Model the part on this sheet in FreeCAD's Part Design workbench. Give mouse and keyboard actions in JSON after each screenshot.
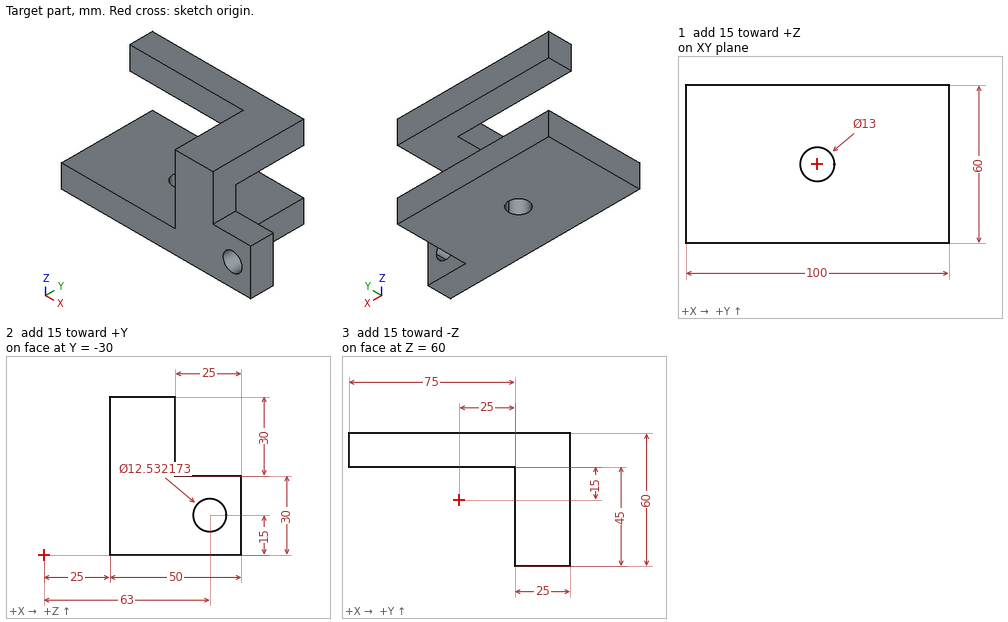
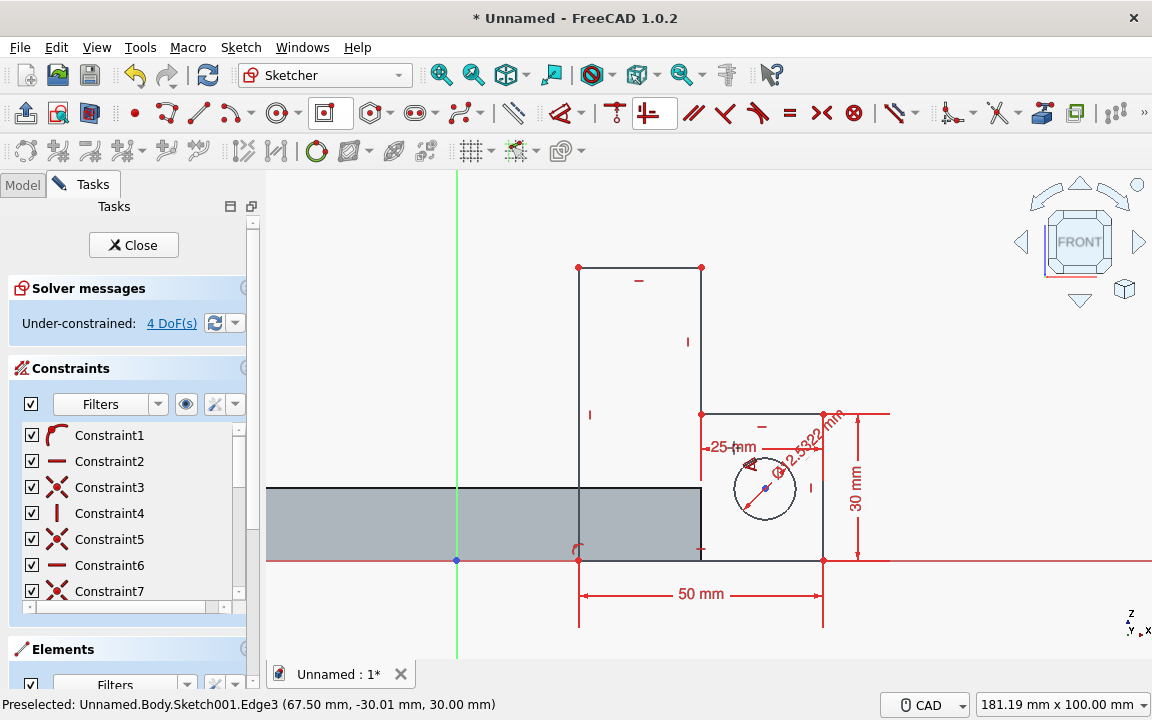
{"action": "left_click", "coordinate": [701, 370]}
{"action": "left_click", "coordinate": [735, 341]}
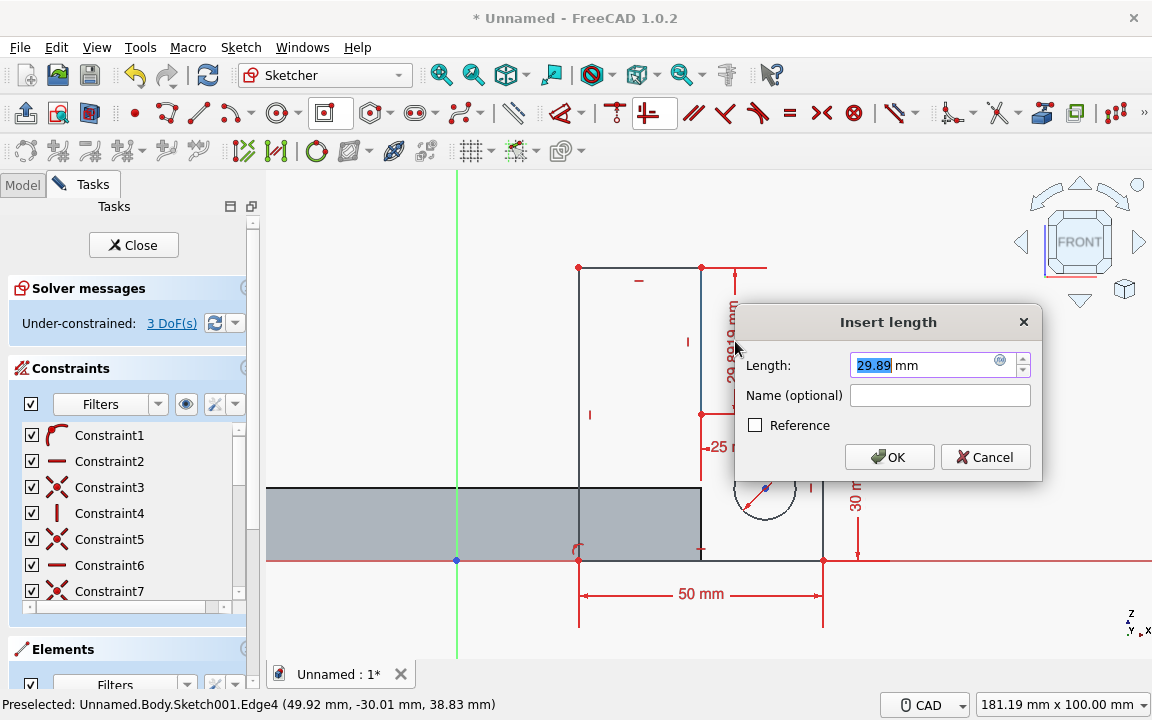
{"action": "type", "text": "30"}
{"action": "key", "text": "Return"}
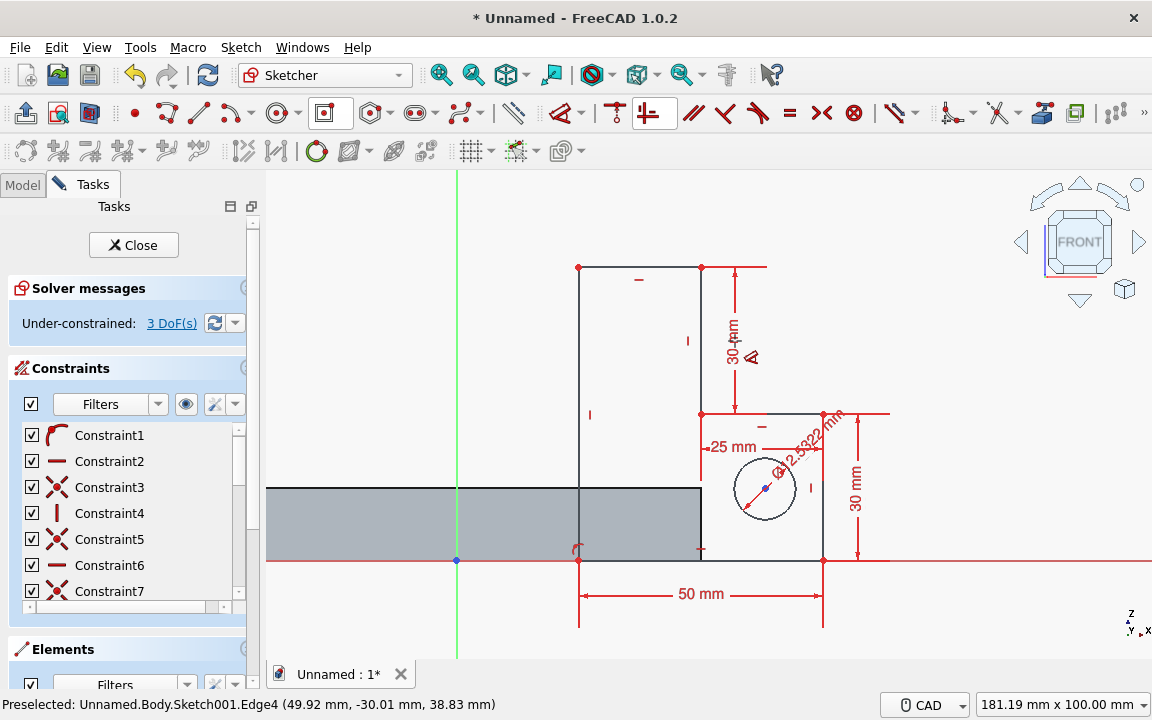
{"action": "left_click", "coordinate": [765, 489]}
{"action": "left_click", "coordinate": [611, 595]}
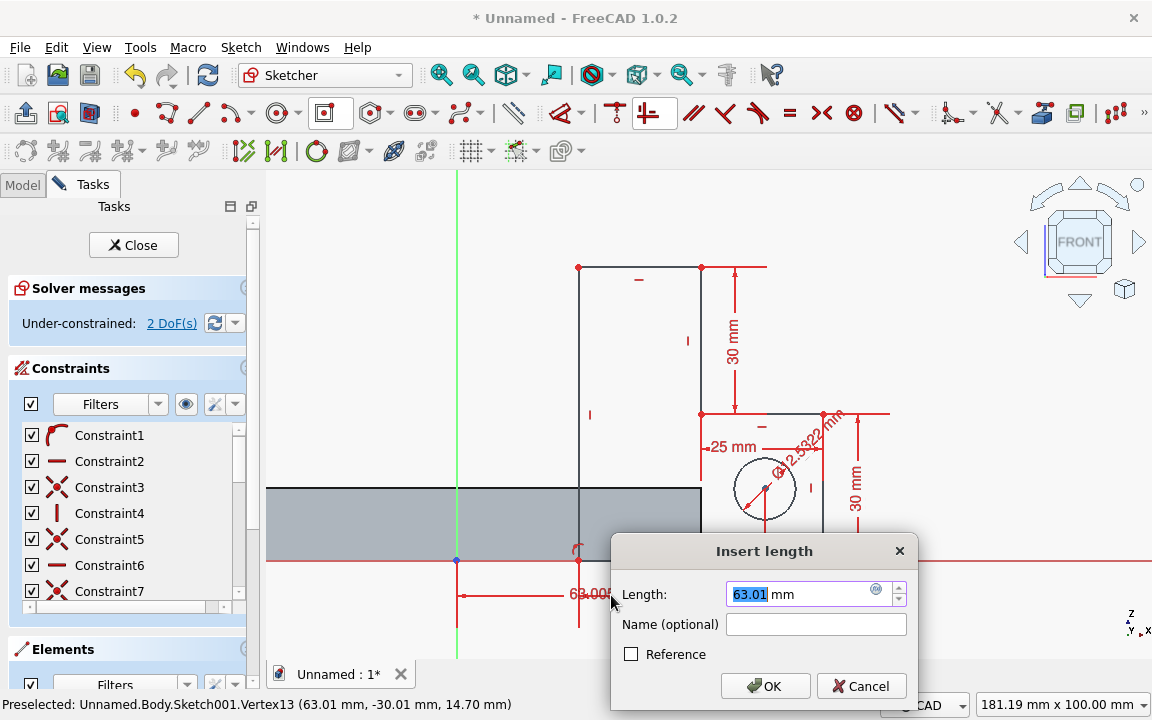
{"action": "type", "text": "63"}
{"action": "key", "text": "Return"}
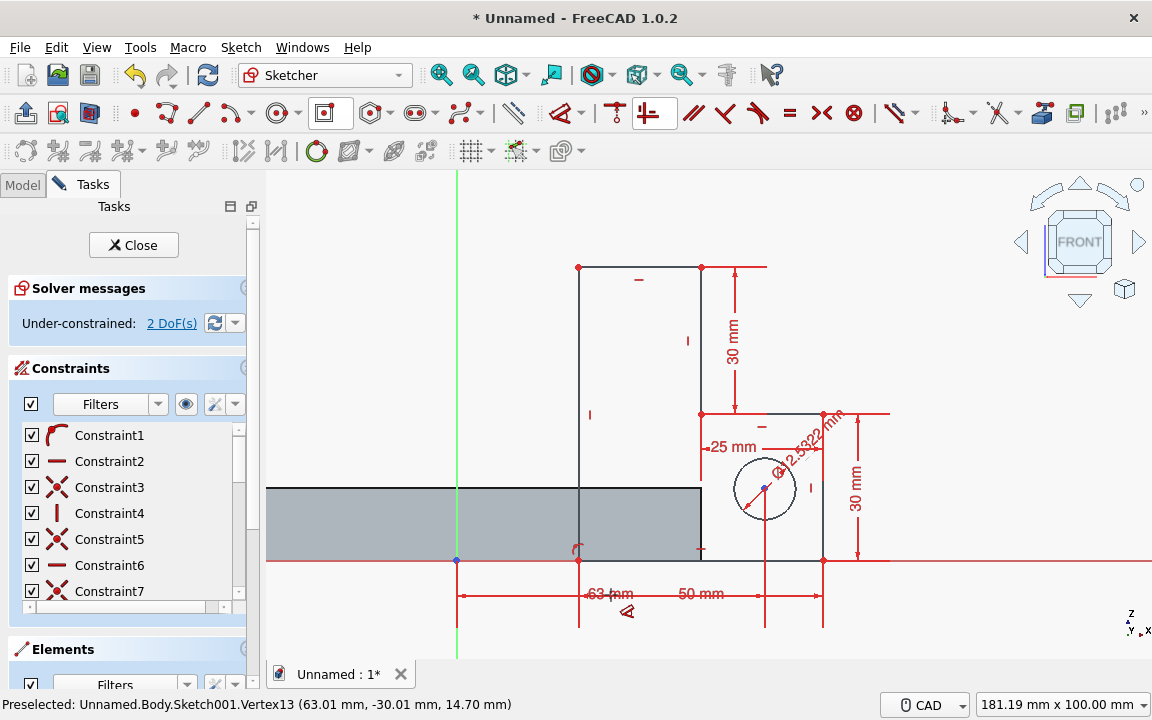
{"action": "left_click", "coordinate": [765, 489]}
{"action": "left_click", "coordinate": [423, 525]}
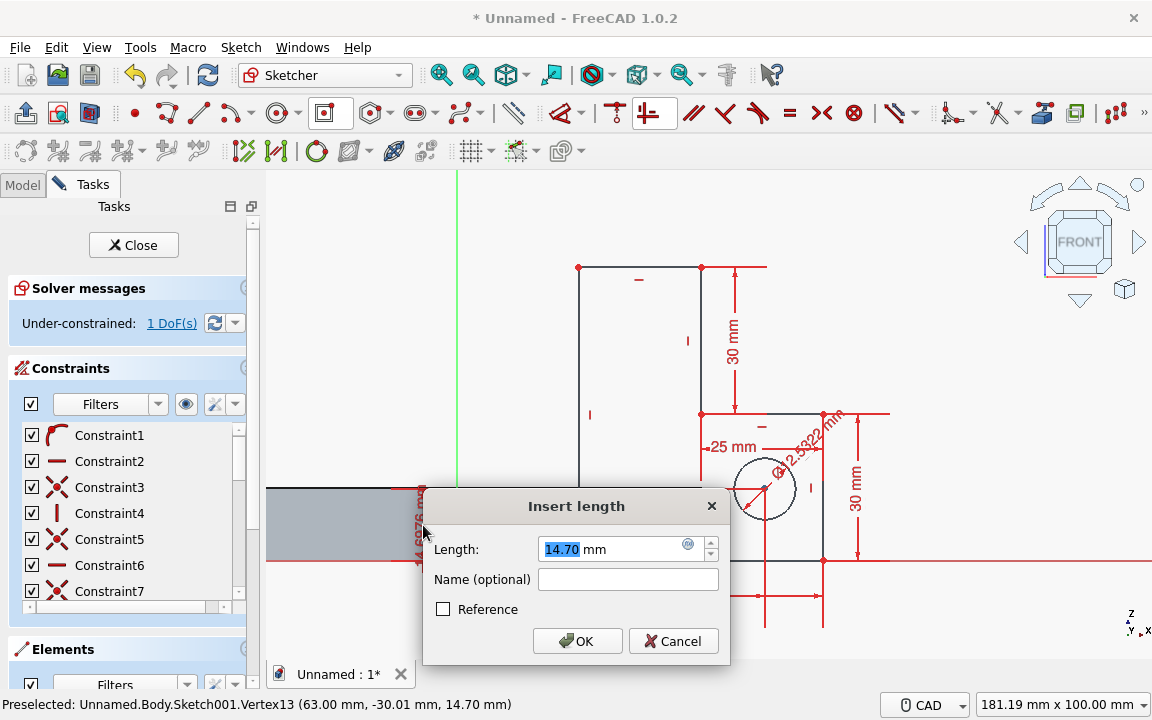
{"action": "type", "text": "15"}
{"action": "key", "text": "Return"}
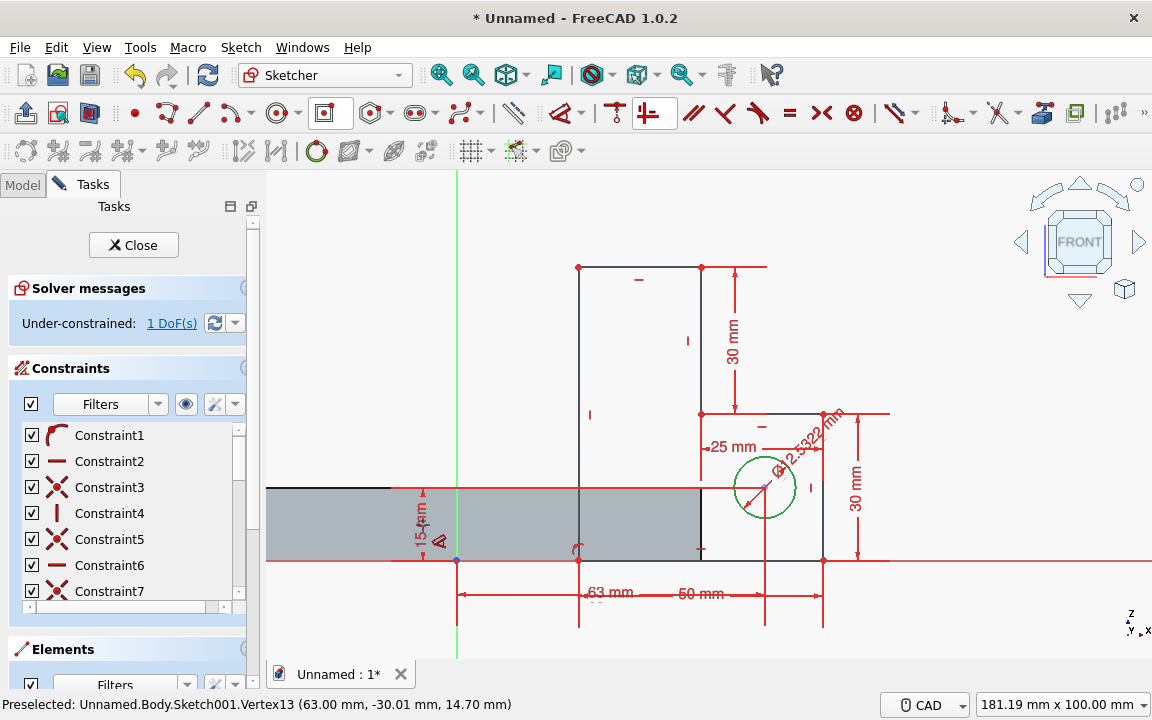
{"action": "left_click", "coordinate": [579, 561]}
{"action": "left_click", "coordinate": [518, 595]}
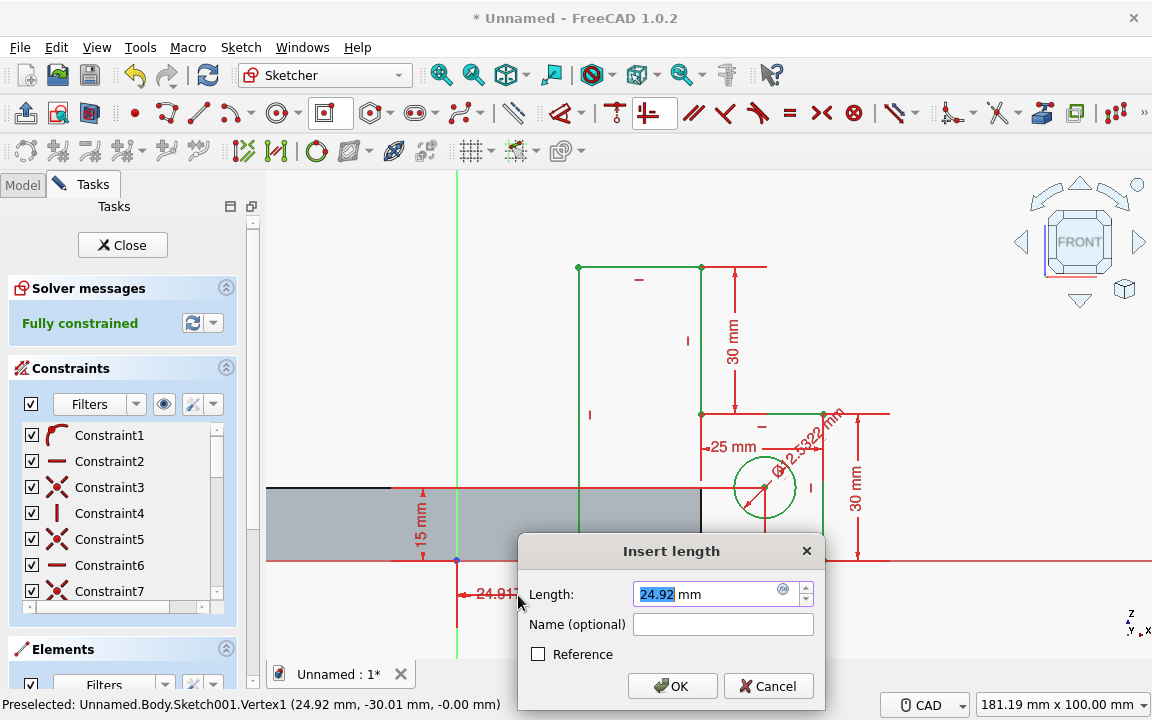
{"action": "type", "text": "25"}
{"action": "key", "text": "Return"}
{"action": "key", "text": "Escape"}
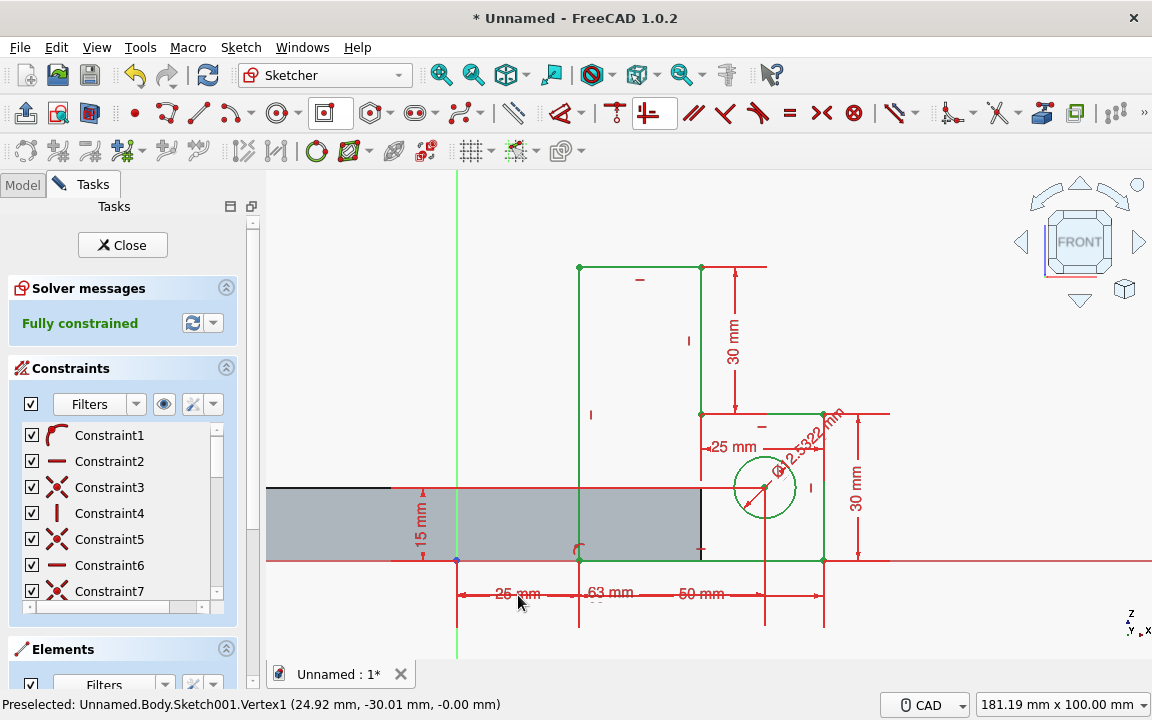
{"action": "left_click", "coordinate": [123, 245]}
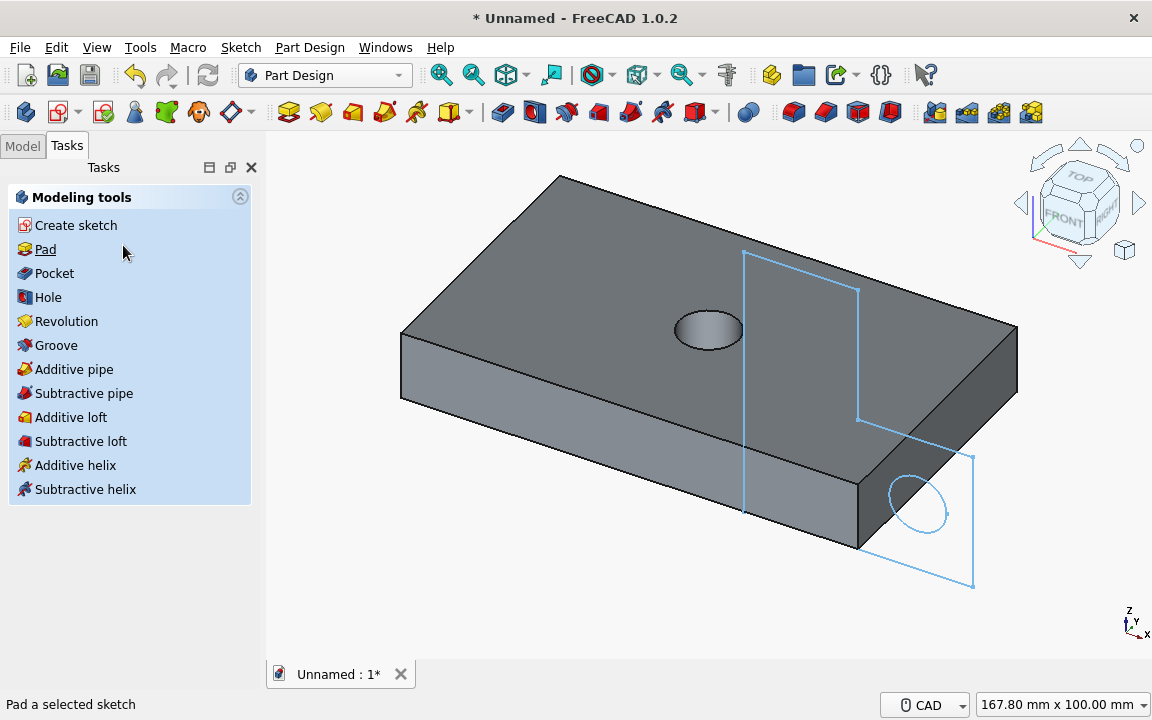
{"action": "left_click", "coordinate": [290, 112]}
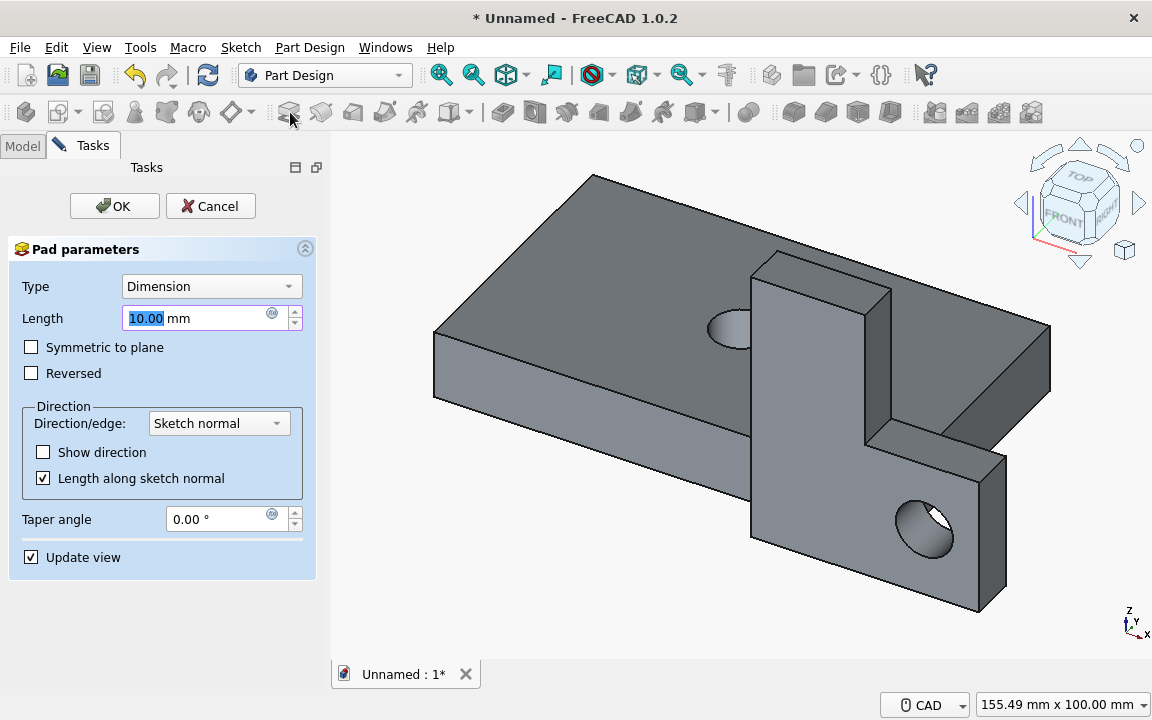
{"action": "type", "text": "15"}
{"action": "key", "text": "Tab"}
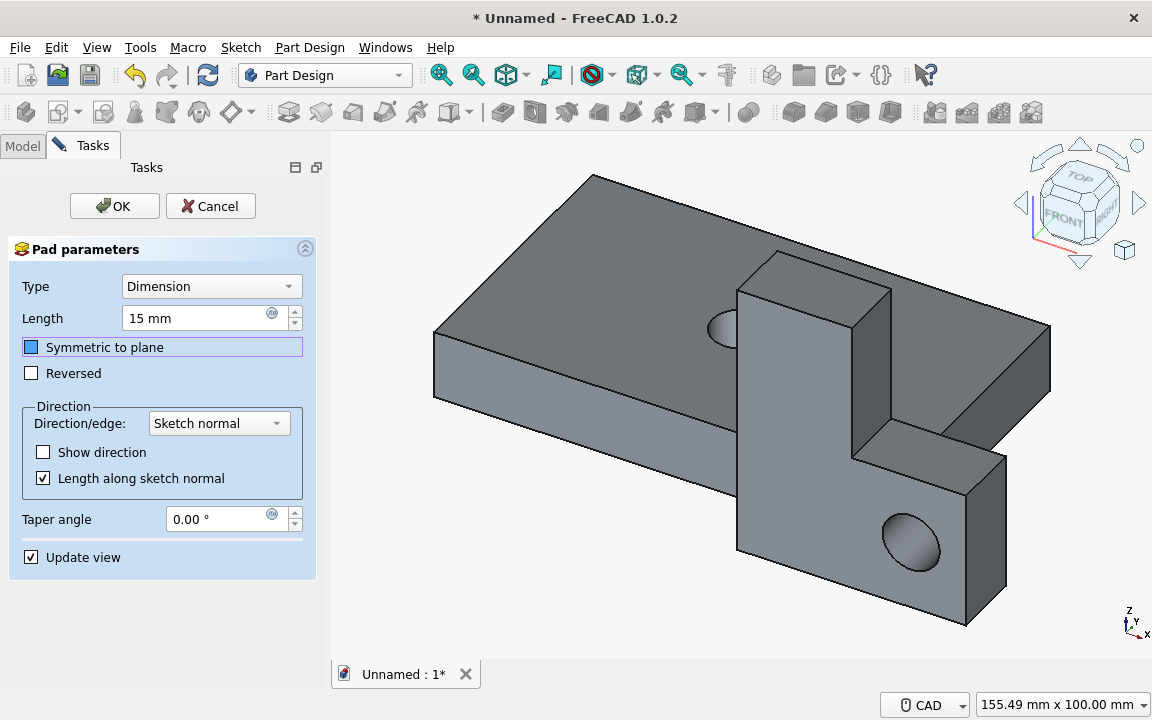
{"action": "left_click", "coordinate": [30, 373]}